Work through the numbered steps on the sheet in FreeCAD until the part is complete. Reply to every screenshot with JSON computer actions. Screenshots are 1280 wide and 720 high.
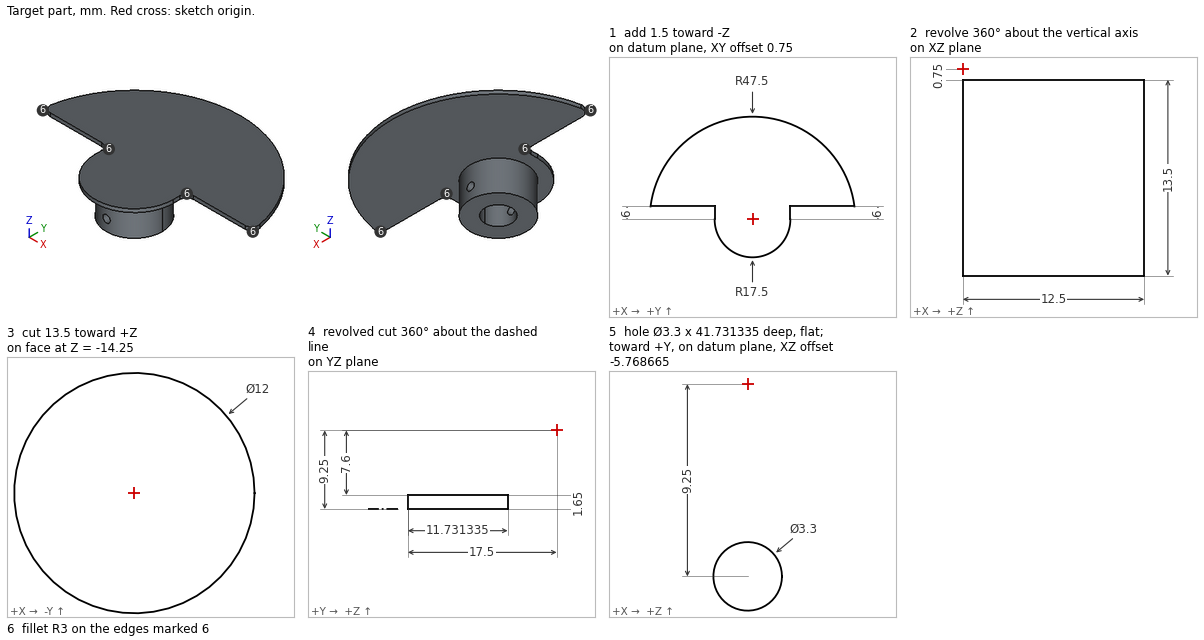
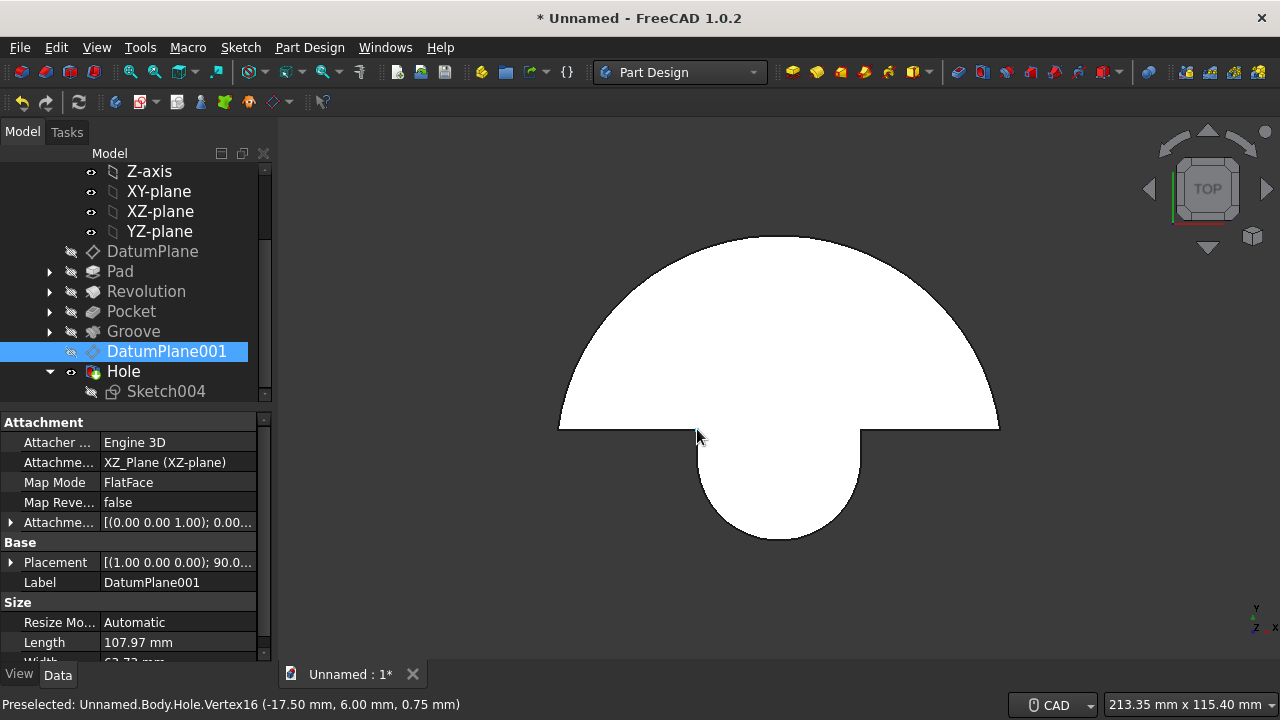
{"action": "key", "text": "1"}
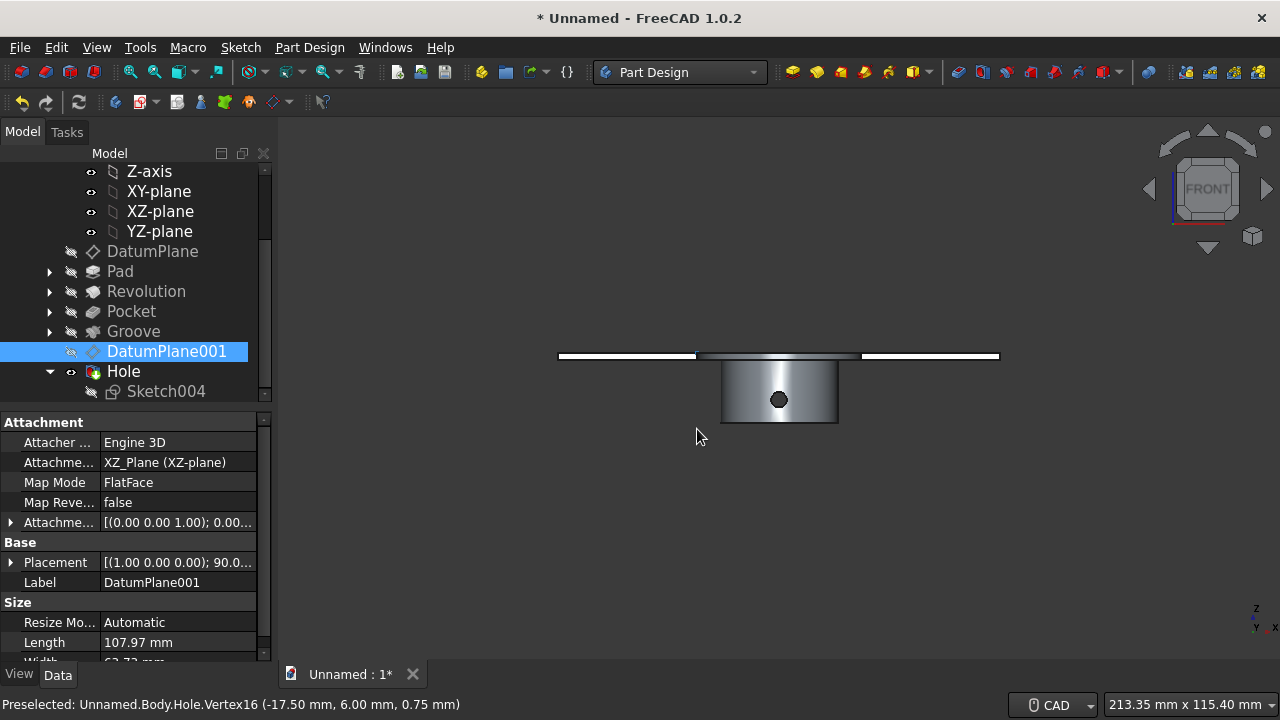
{"action": "key", "text": "v f"}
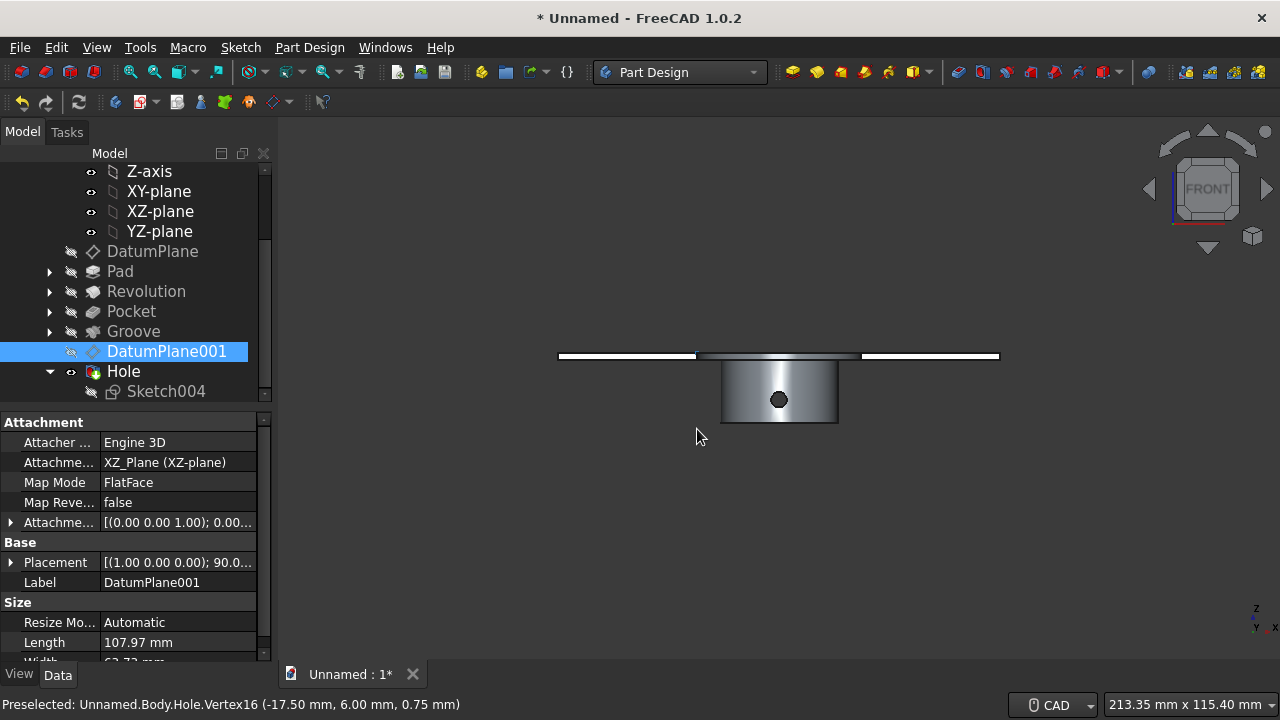
{"action": "scroll", "coordinate": [697, 355], "scroll_direction": "up", "scroll_amount": 9}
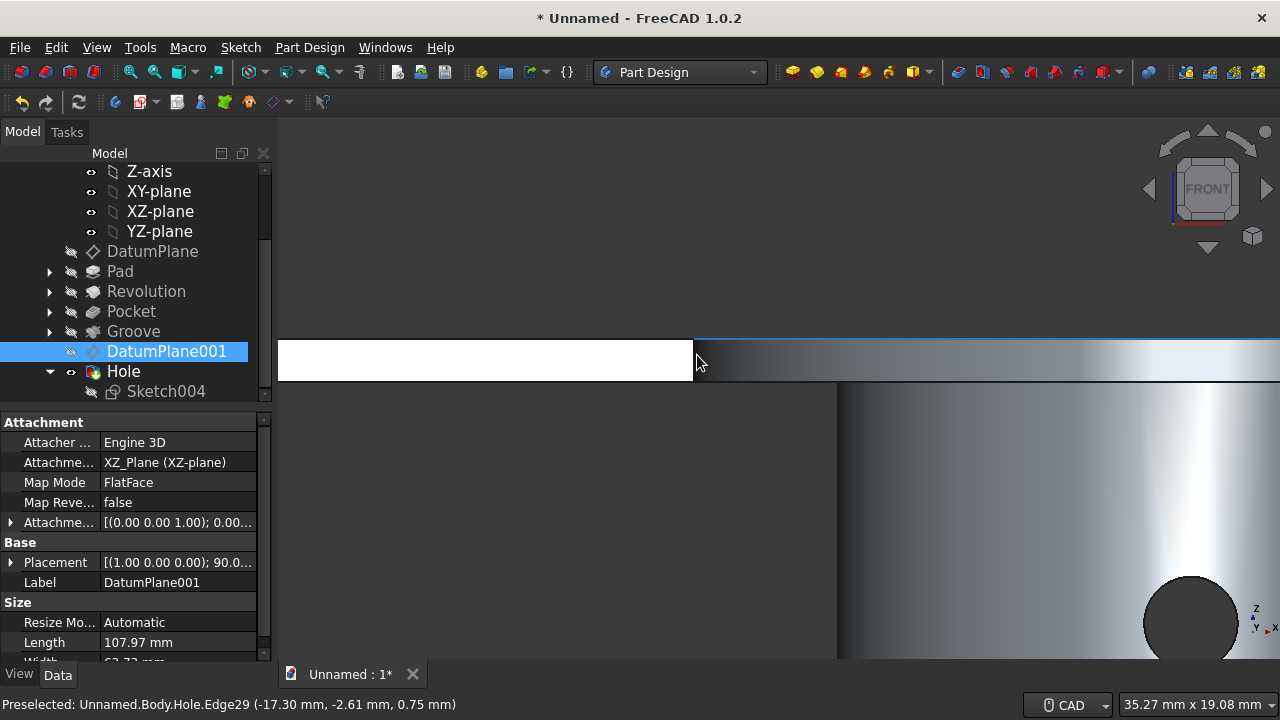
{"action": "key", "text": "v f"}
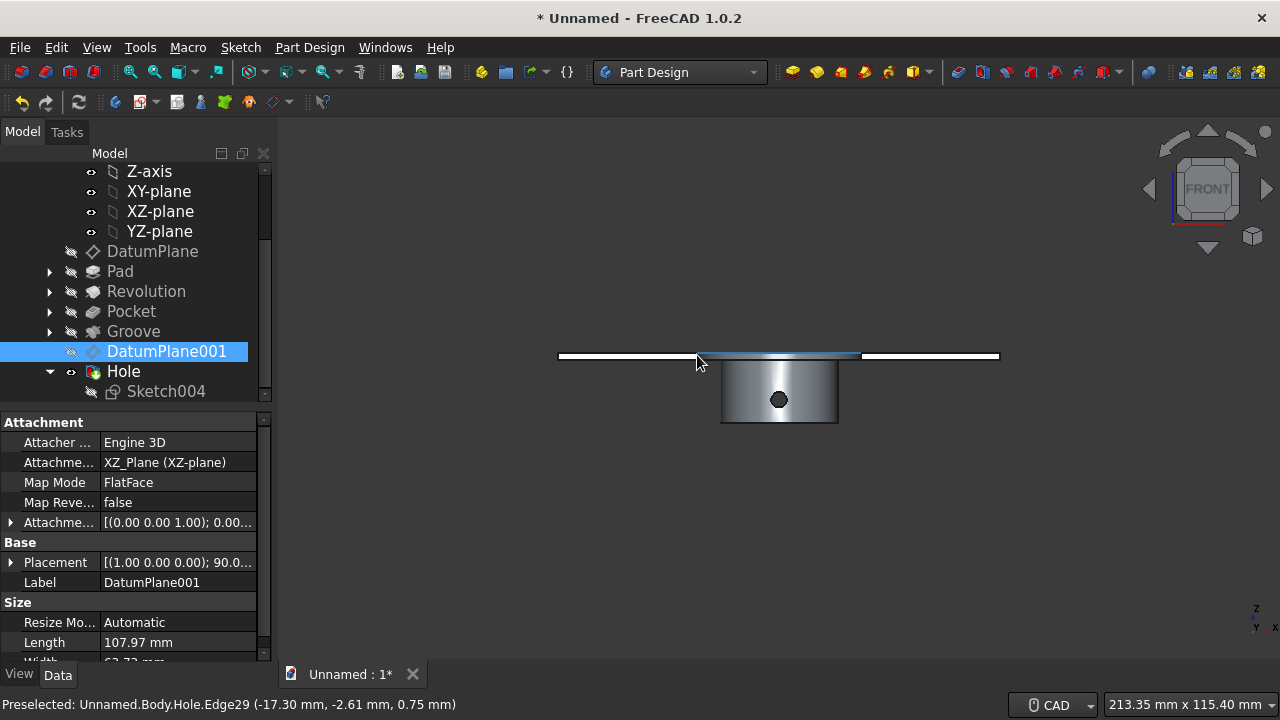
{"action": "key", "text": "3"}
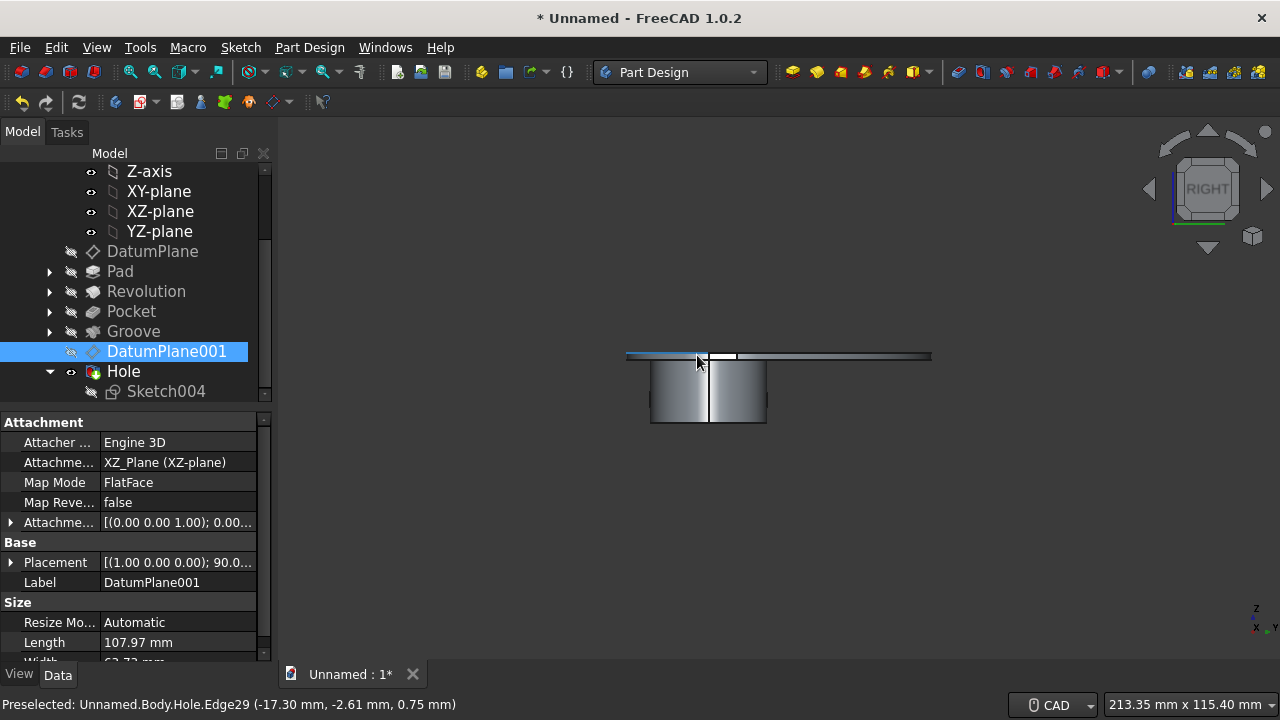
{"action": "left_click", "coordinate": [132, 72]}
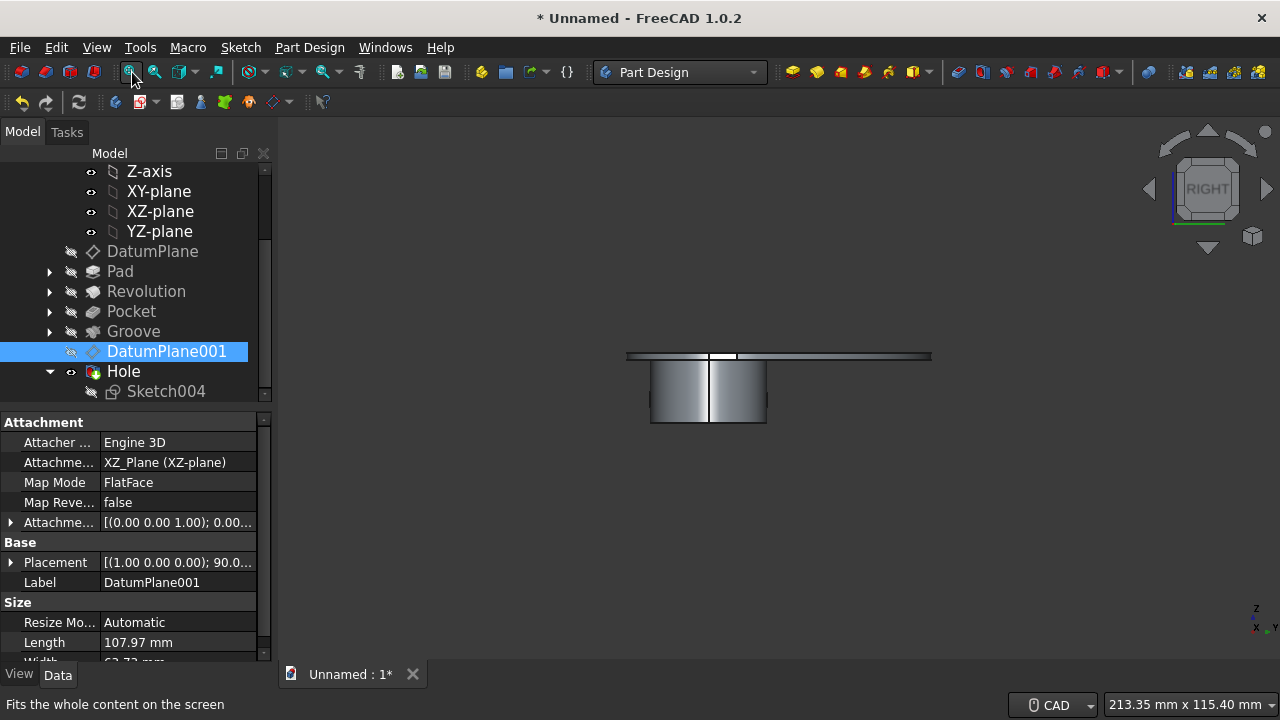
{"action": "scroll", "coordinate": [737, 355], "scroll_direction": "up", "scroll_amount": 9}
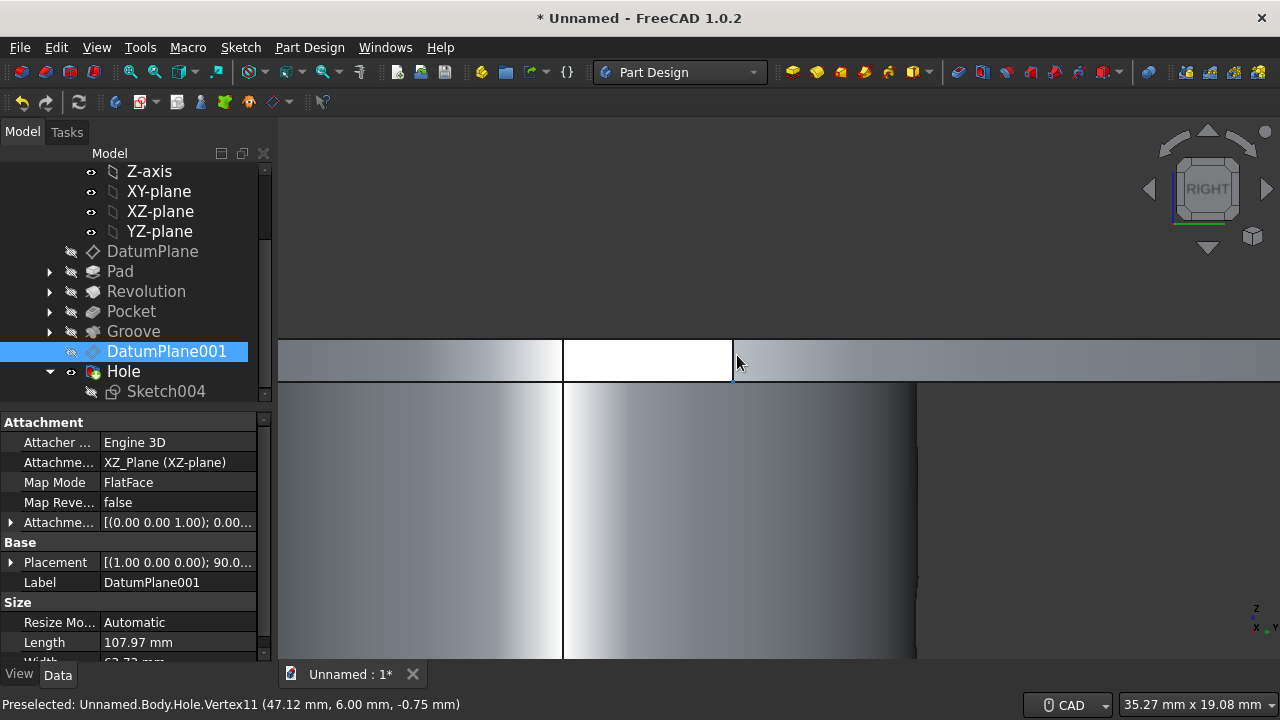
{"action": "left_click", "coordinate": [733, 360]}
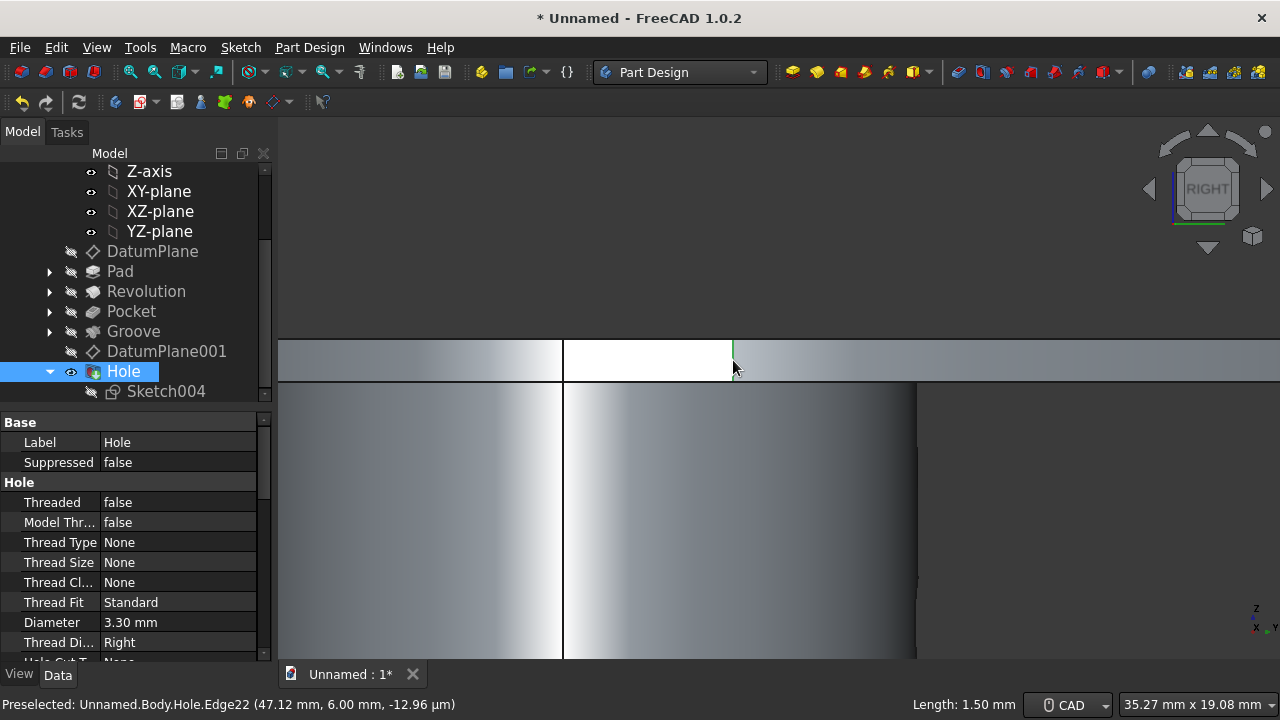
{"action": "left_click", "coordinate": [132, 72]}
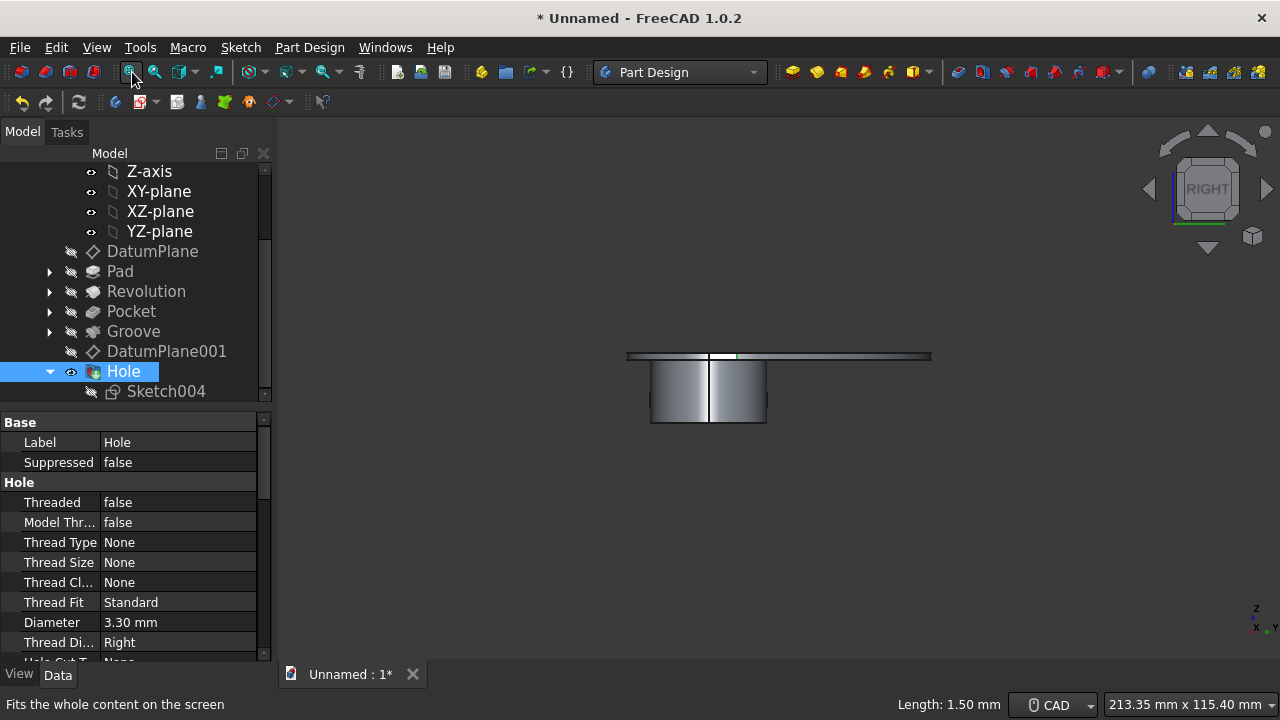
{"action": "key", "text": "5"}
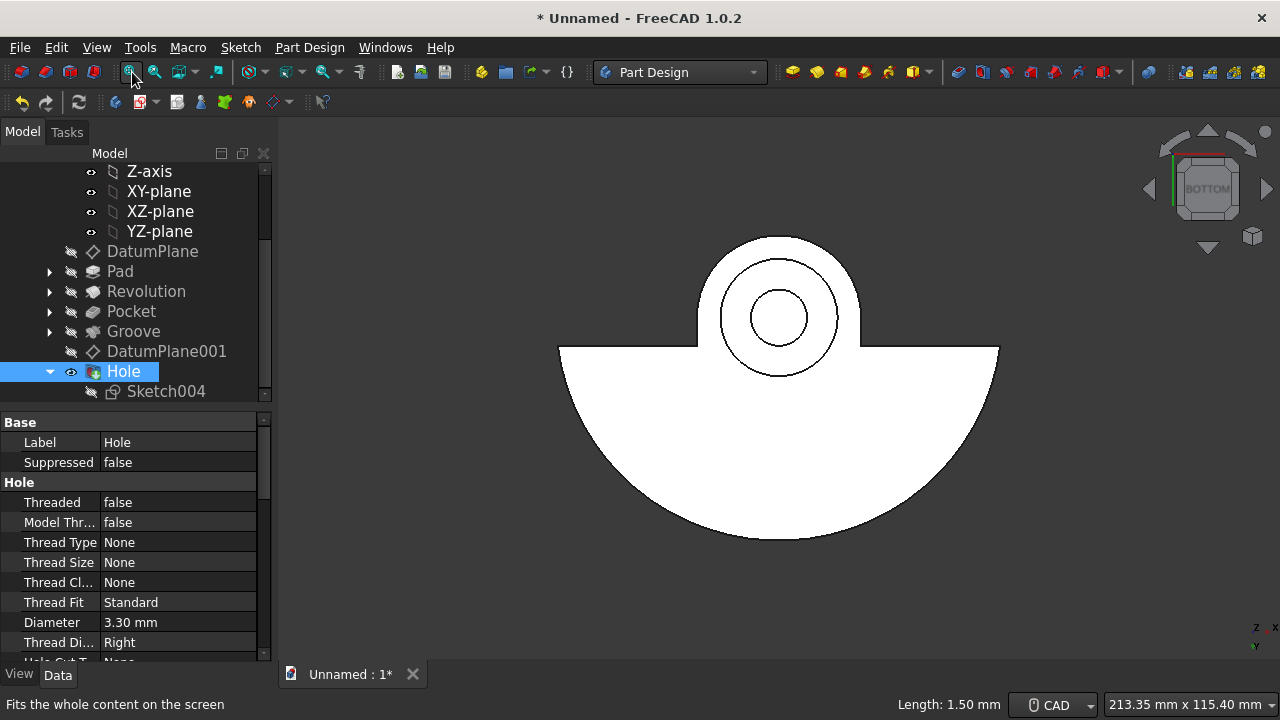
{"action": "scroll", "coordinate": [697, 345], "scroll_direction": "up", "scroll_amount": 9}